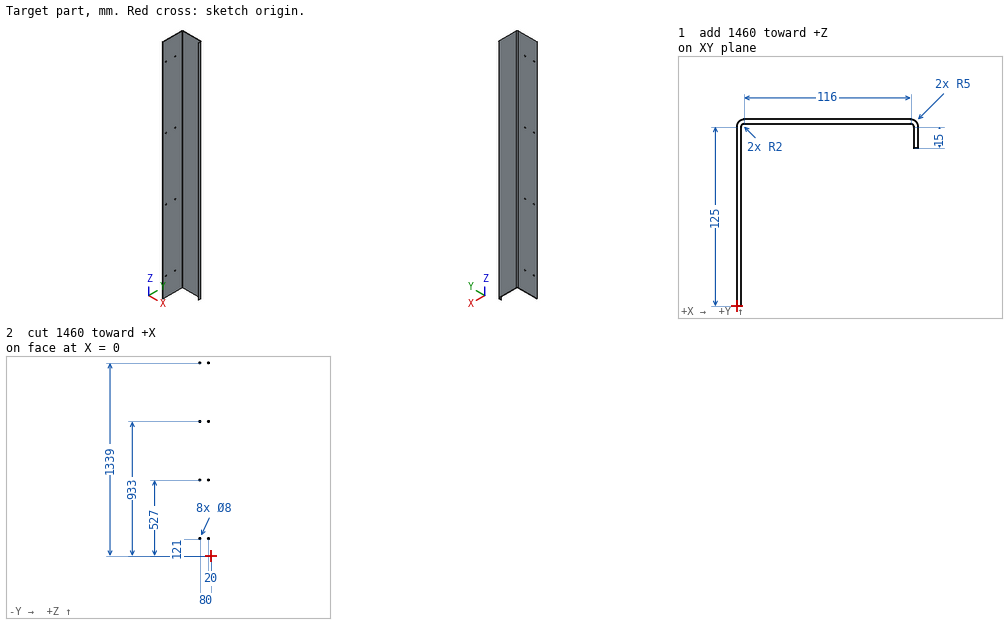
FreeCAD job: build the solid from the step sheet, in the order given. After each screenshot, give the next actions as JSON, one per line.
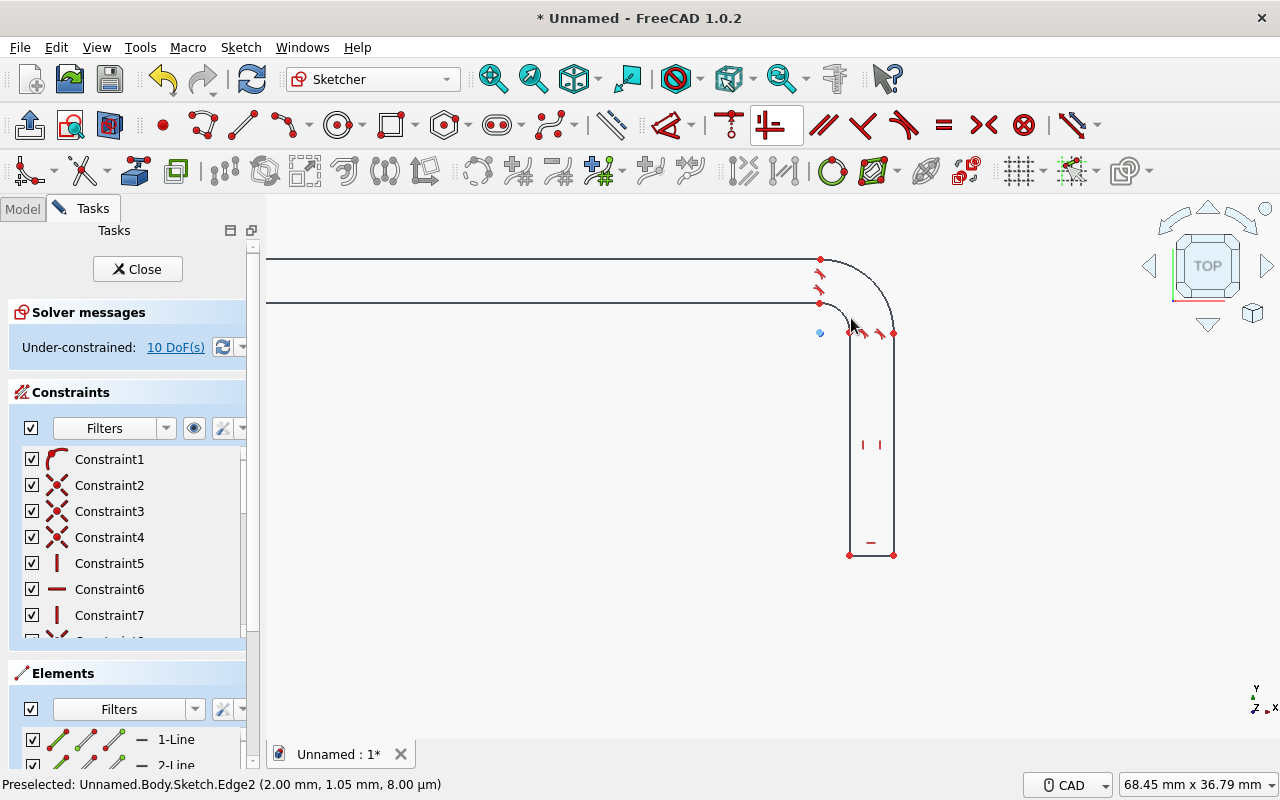
{"action": "left_click", "coordinate": [847, 319]}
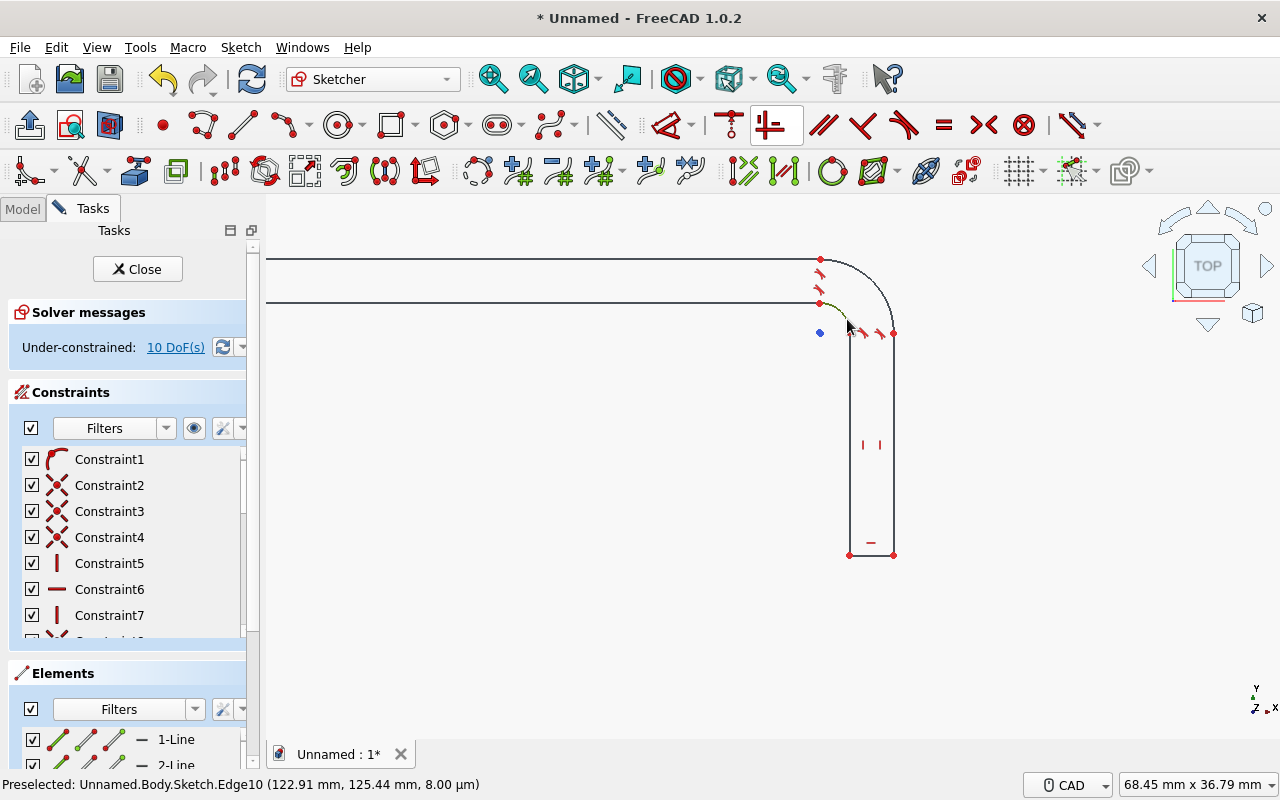
{"action": "left_click", "coordinate": [886, 300]}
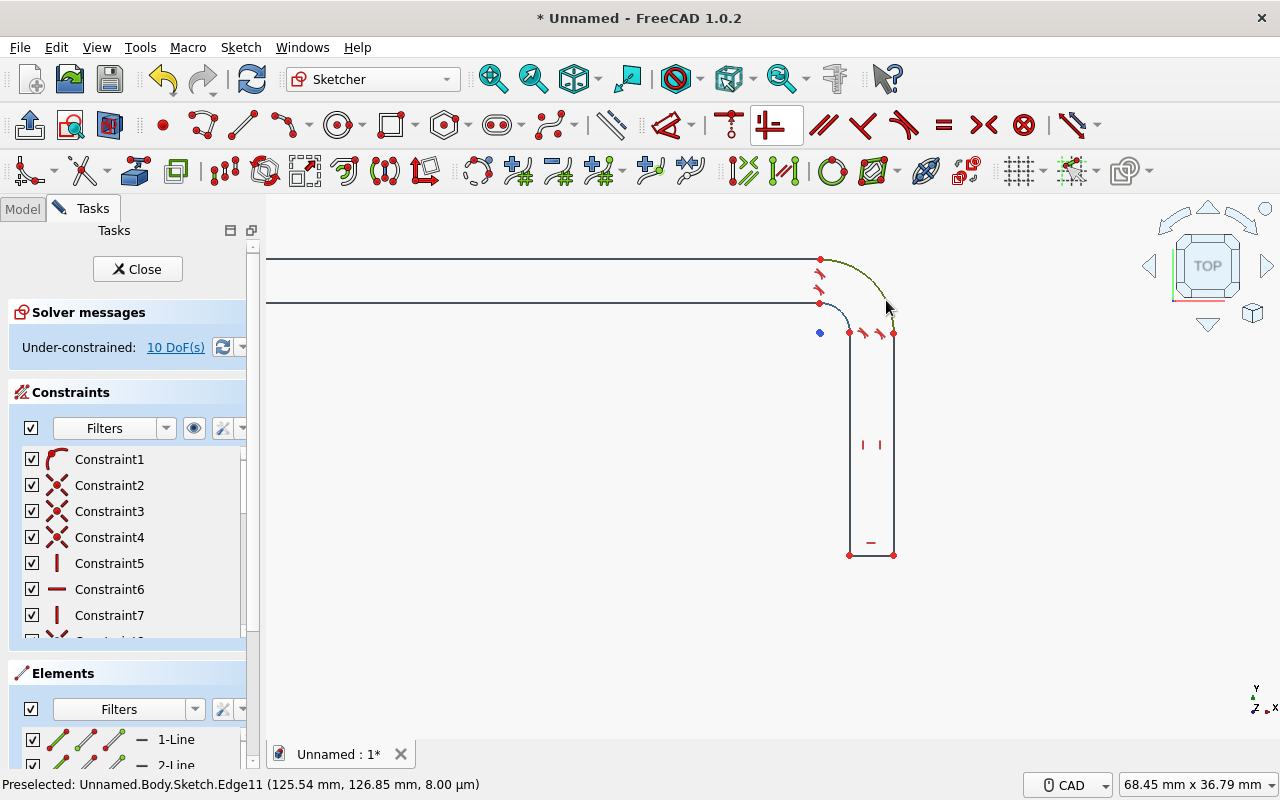
{"action": "key", "text": "c"}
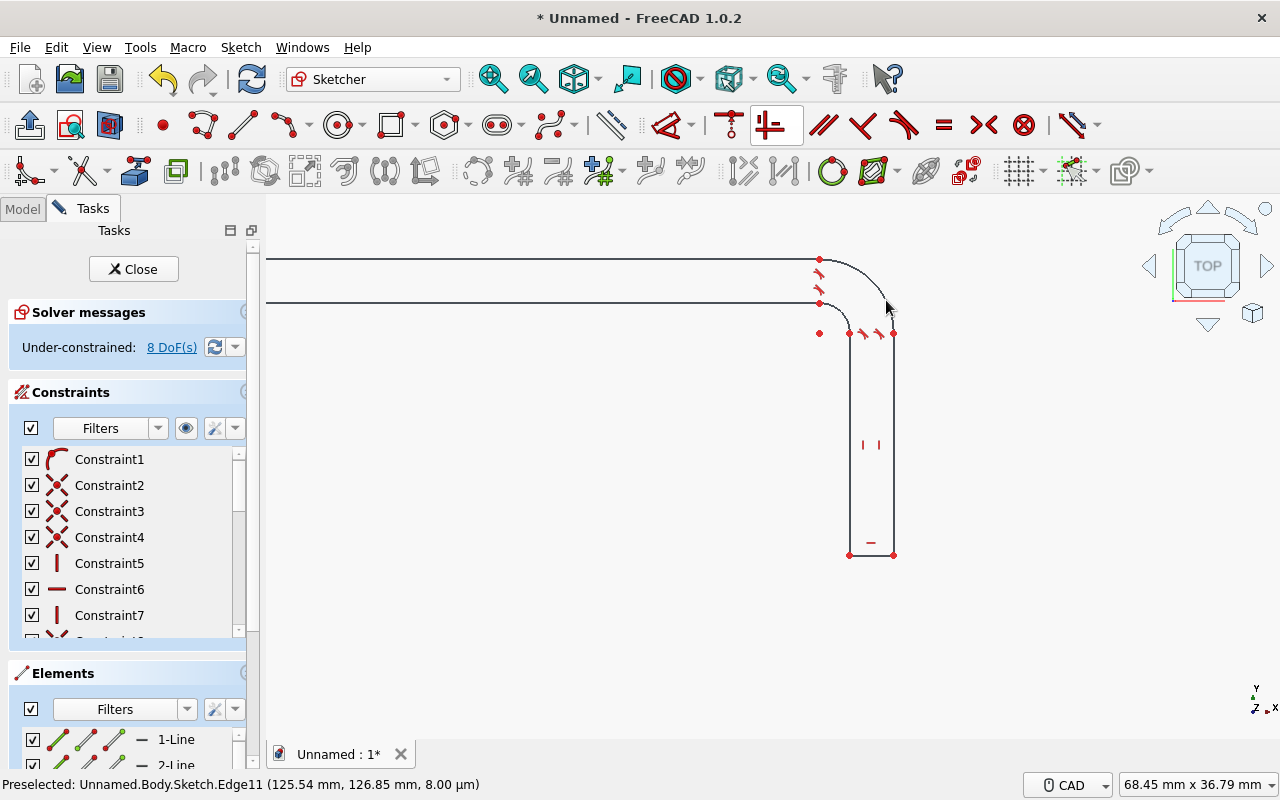
{"action": "scroll", "coordinate": [852, 317], "scroll_direction": "down", "scroll_amount": 9}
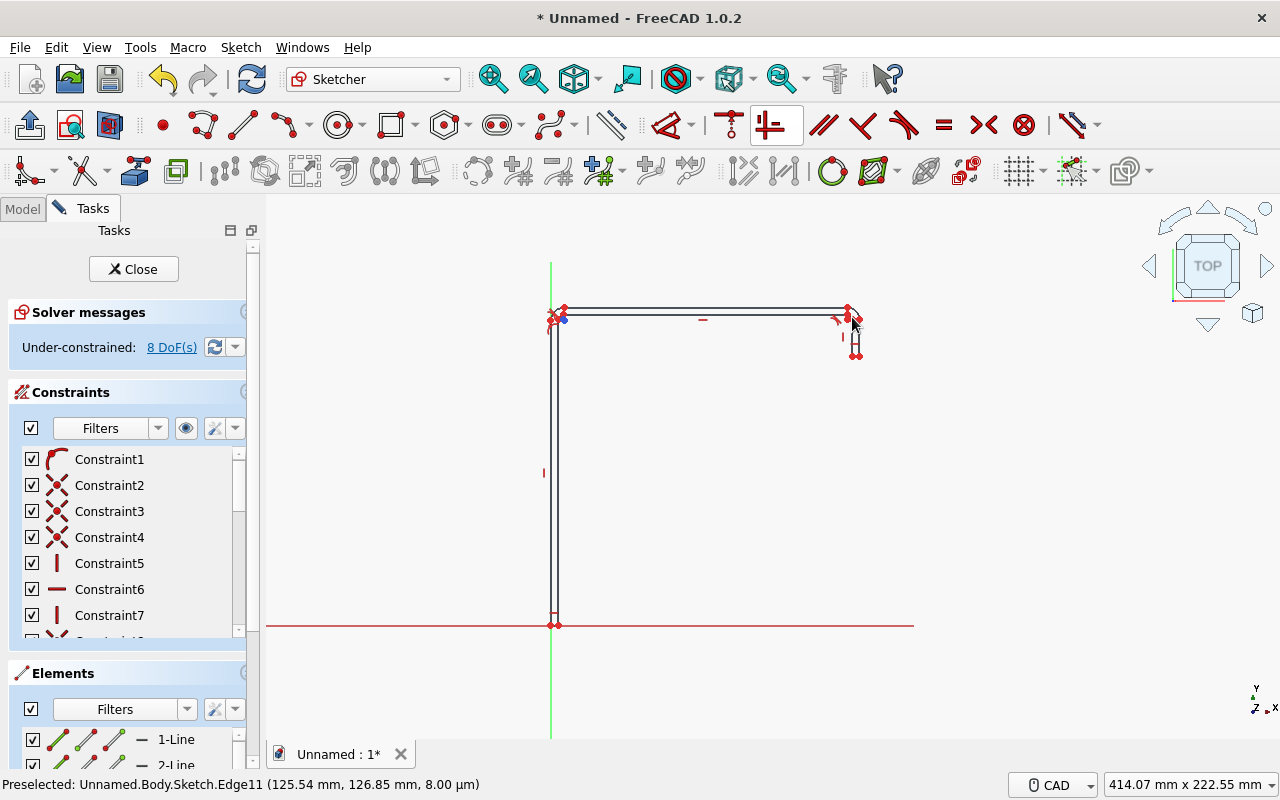
{"action": "scroll", "coordinate": [561, 315], "scroll_direction": "up", "scroll_amount": 9}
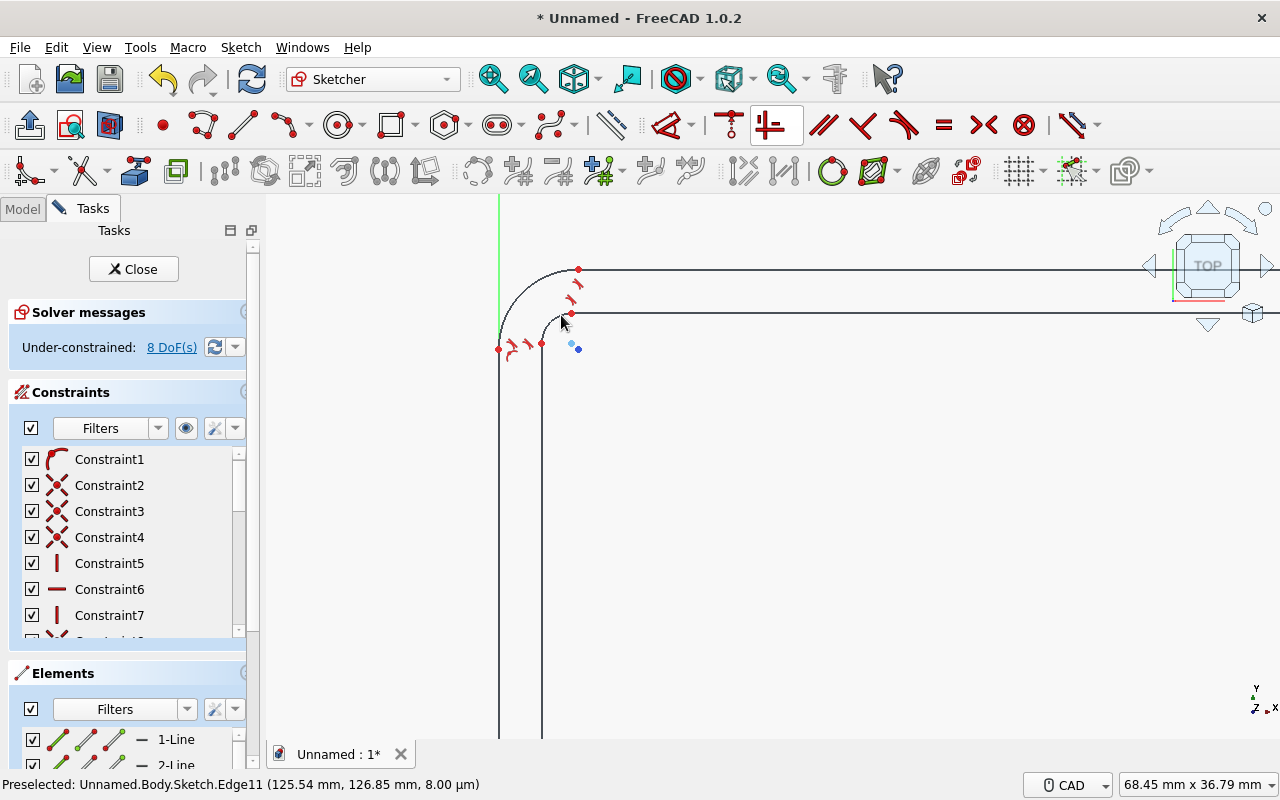
{"action": "left_click", "coordinate": [558, 317]}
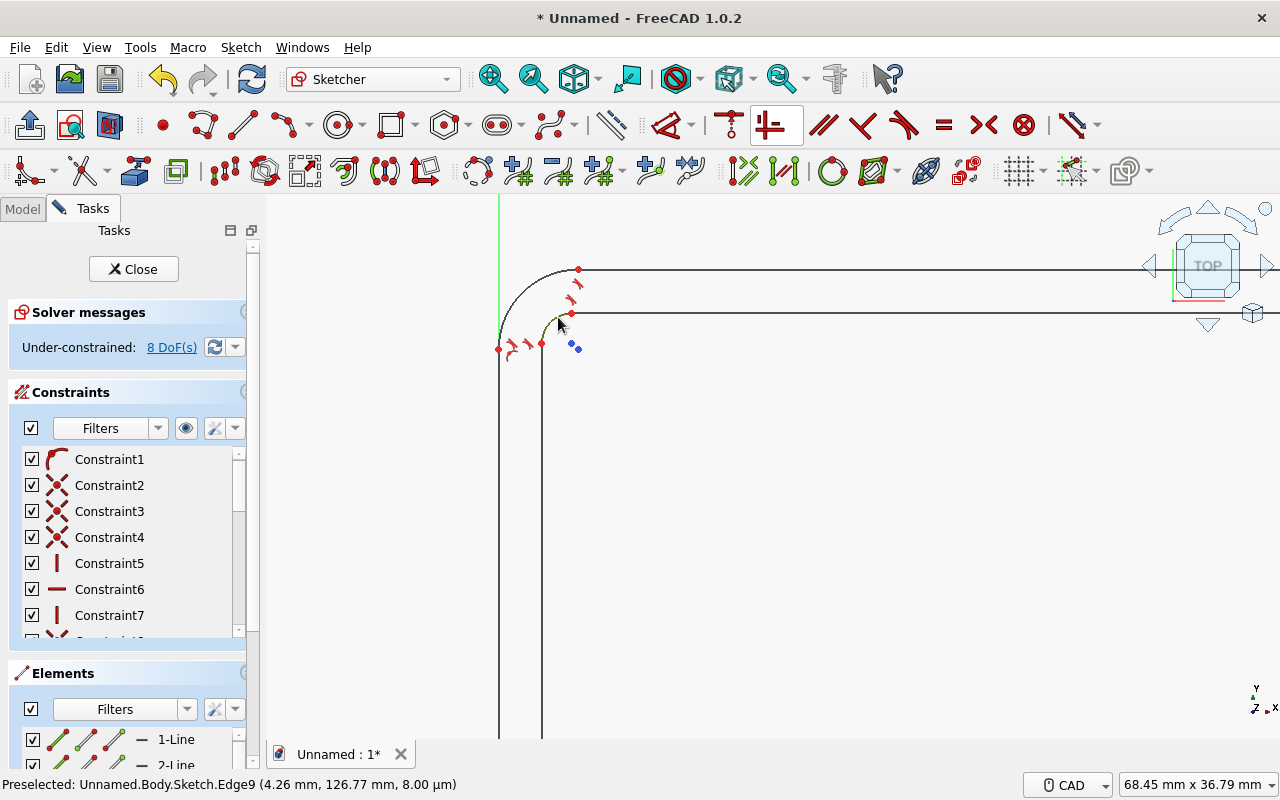
{"action": "left_click", "coordinate": [542, 278]}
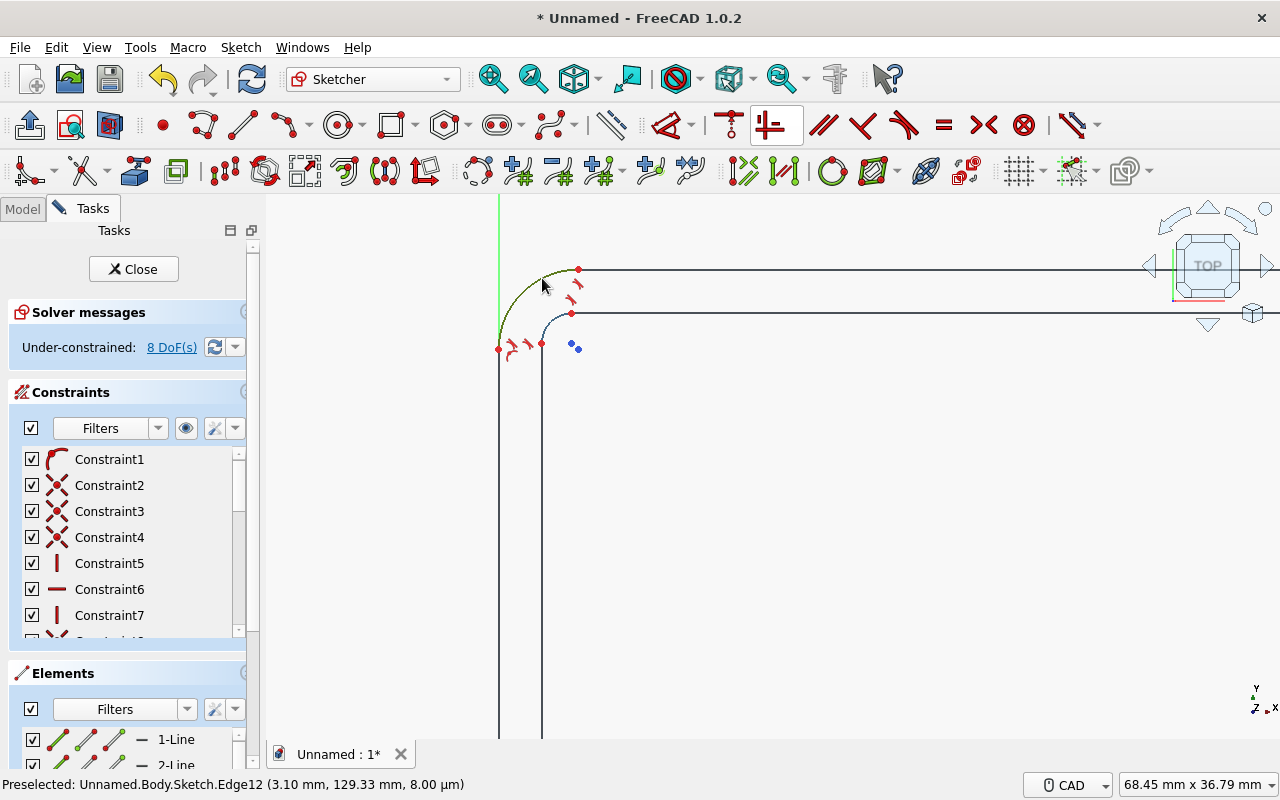
{"action": "left_click", "coordinate": [730, 126]}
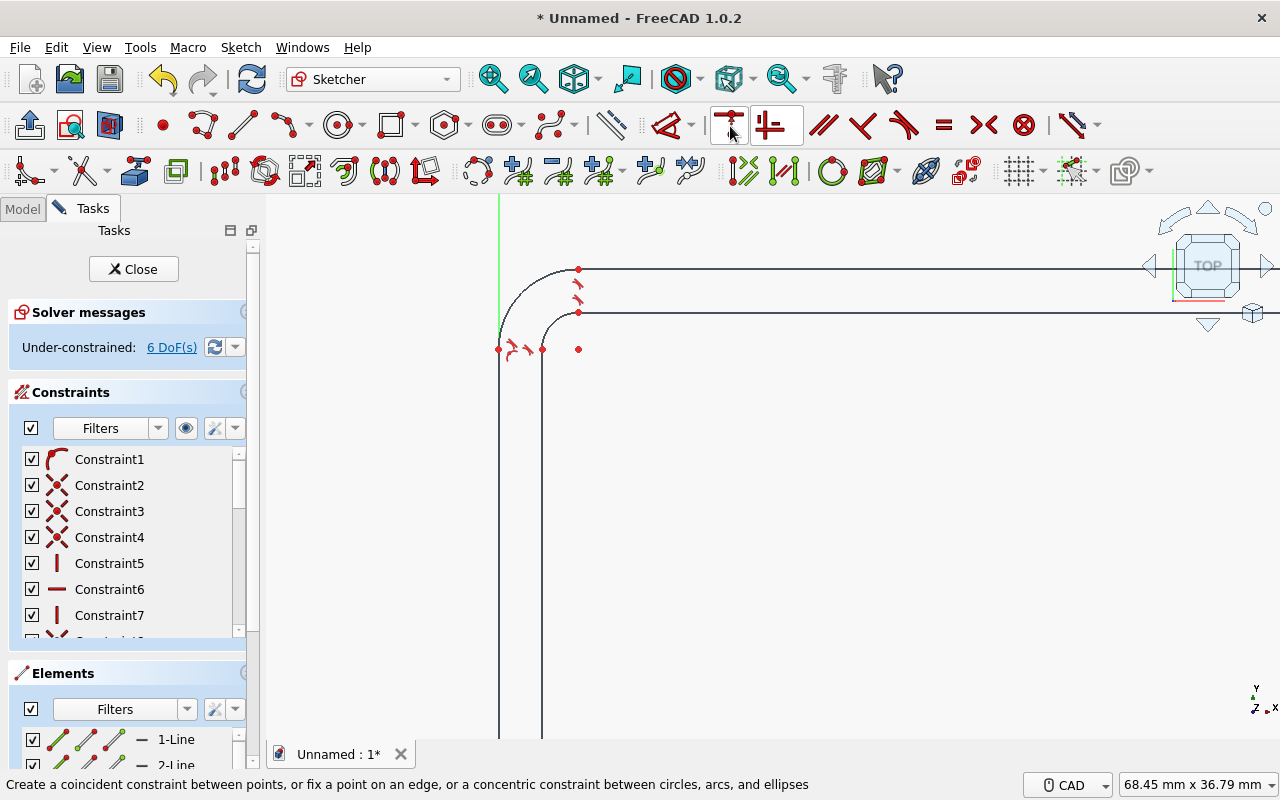
{"action": "left_click", "coordinate": [562, 317]}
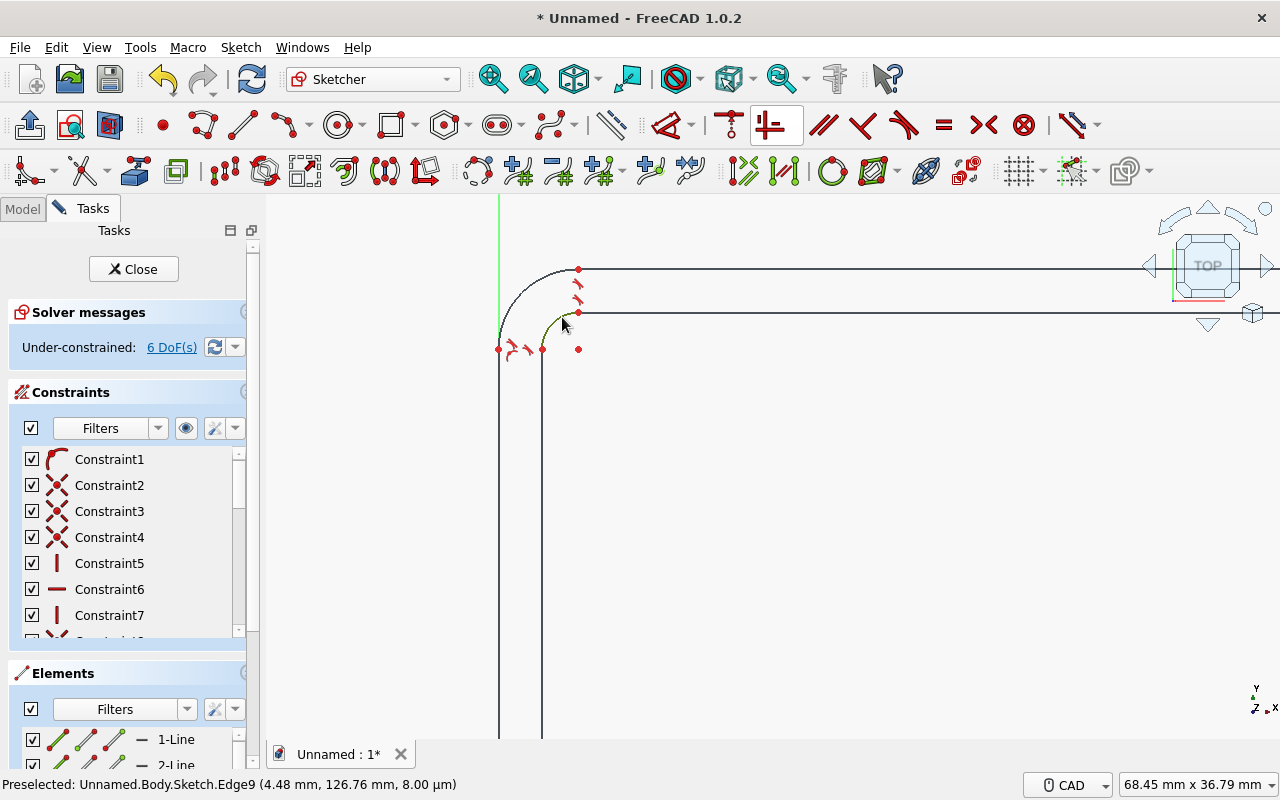
{"action": "scroll", "coordinate": [560, 315], "scroll_direction": "down", "scroll_amount": 9}